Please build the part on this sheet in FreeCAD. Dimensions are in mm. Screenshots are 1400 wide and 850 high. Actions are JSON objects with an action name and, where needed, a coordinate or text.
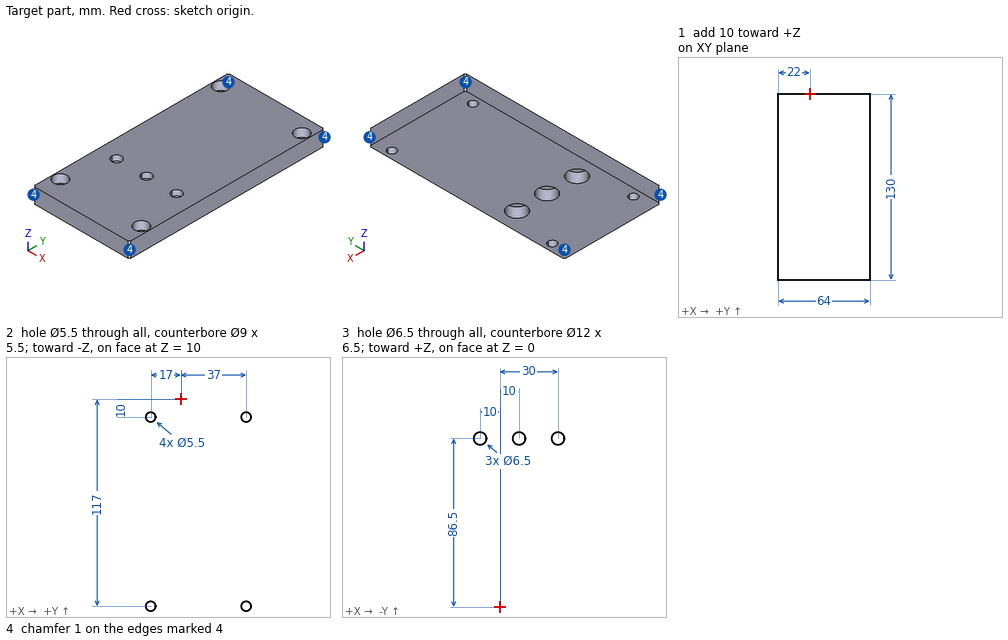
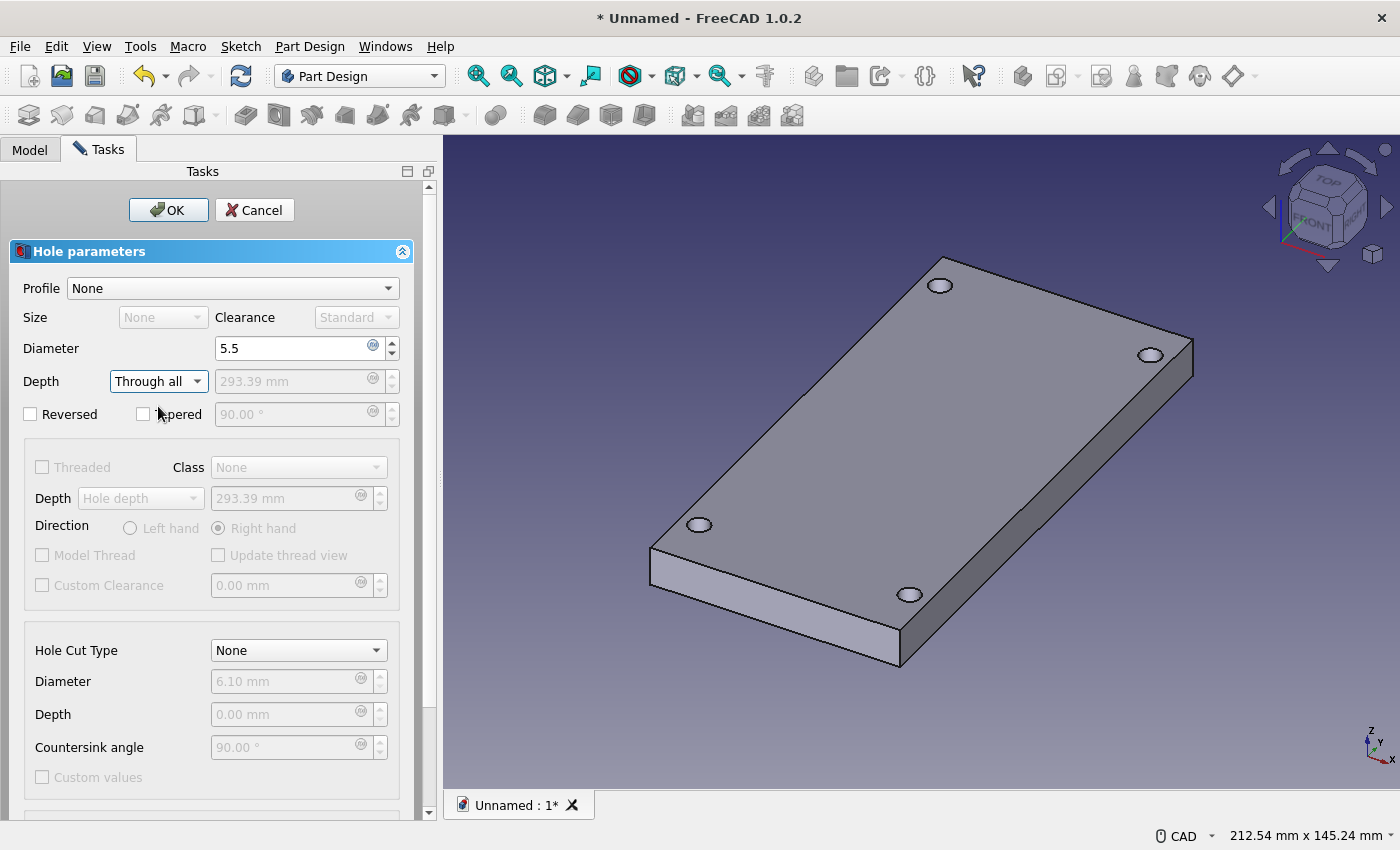
{"action": "left_click", "coordinate": [300, 650]}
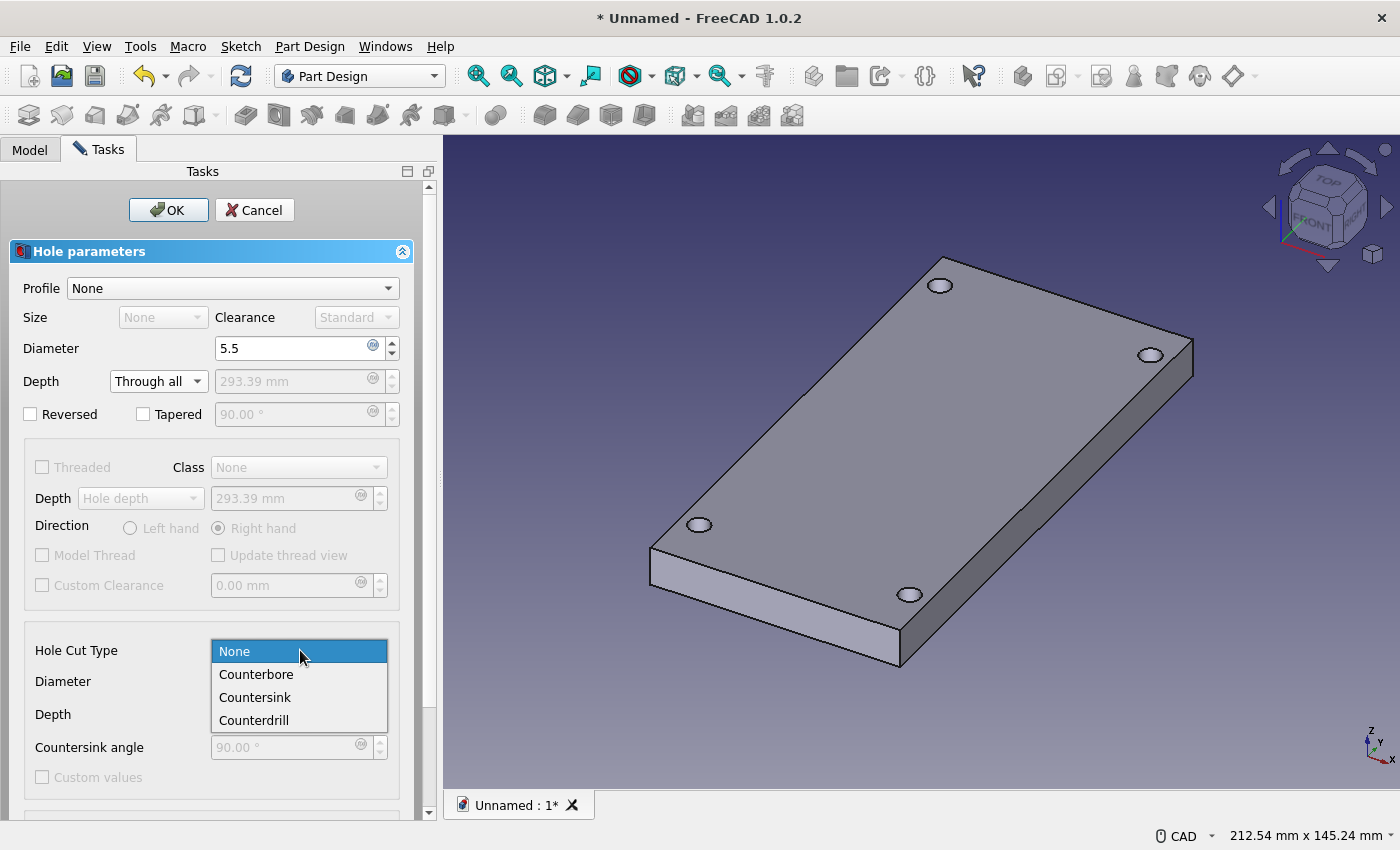
{"action": "left_click", "coordinate": [298, 674]}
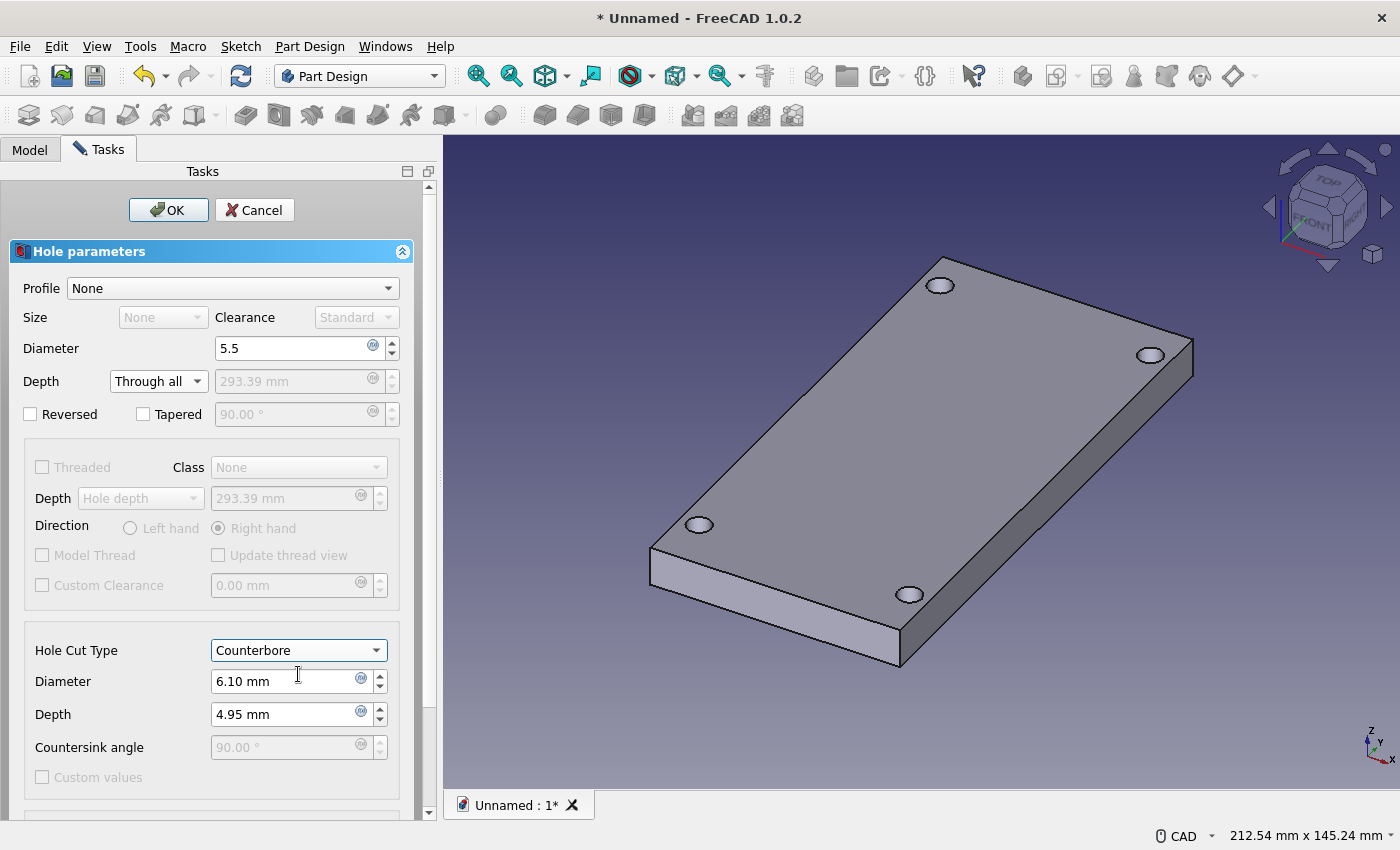
{"action": "triple_click", "coordinate": [292, 682]}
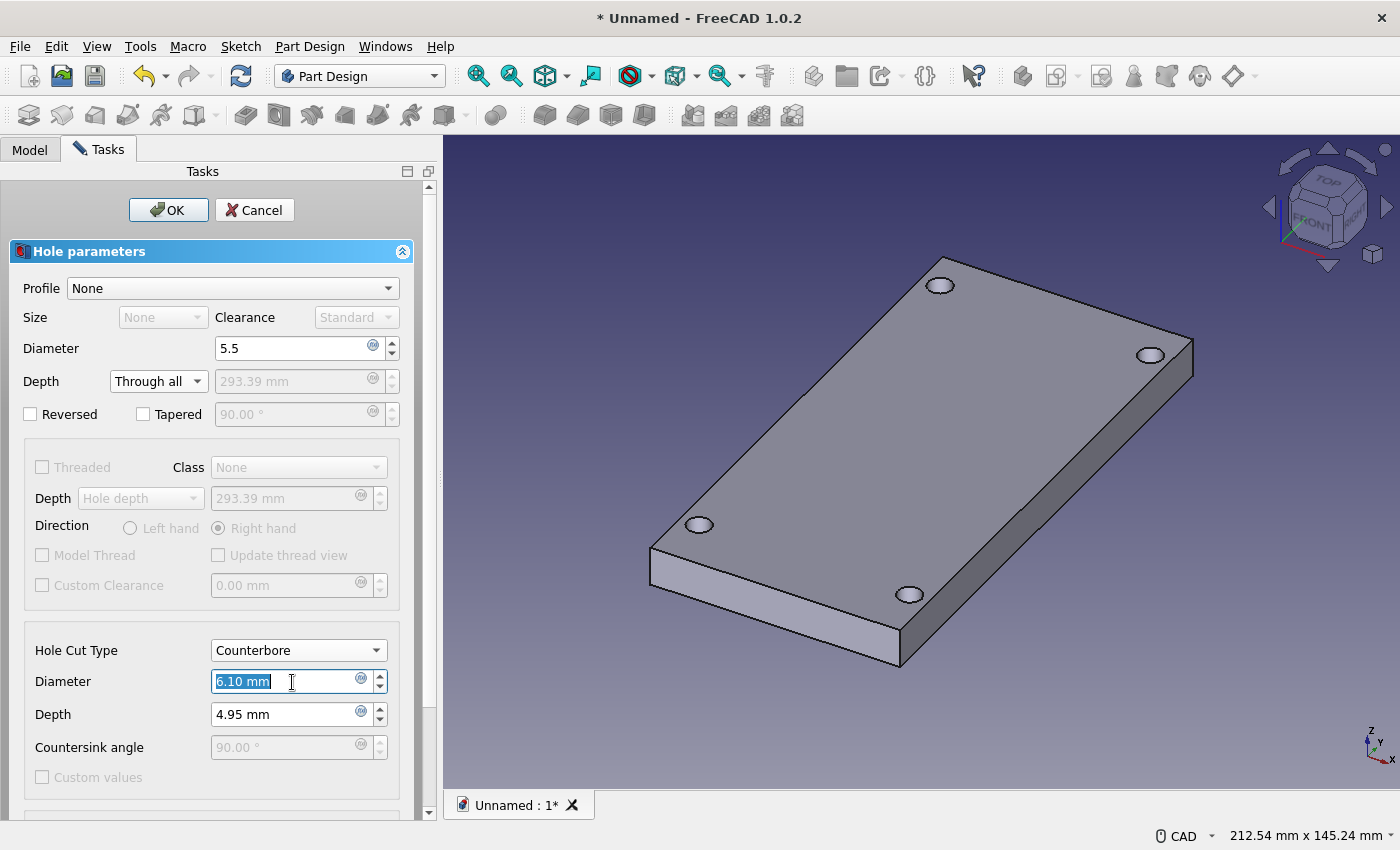
{"action": "type", "text": "9"}
{"action": "key", "text": "Tab"}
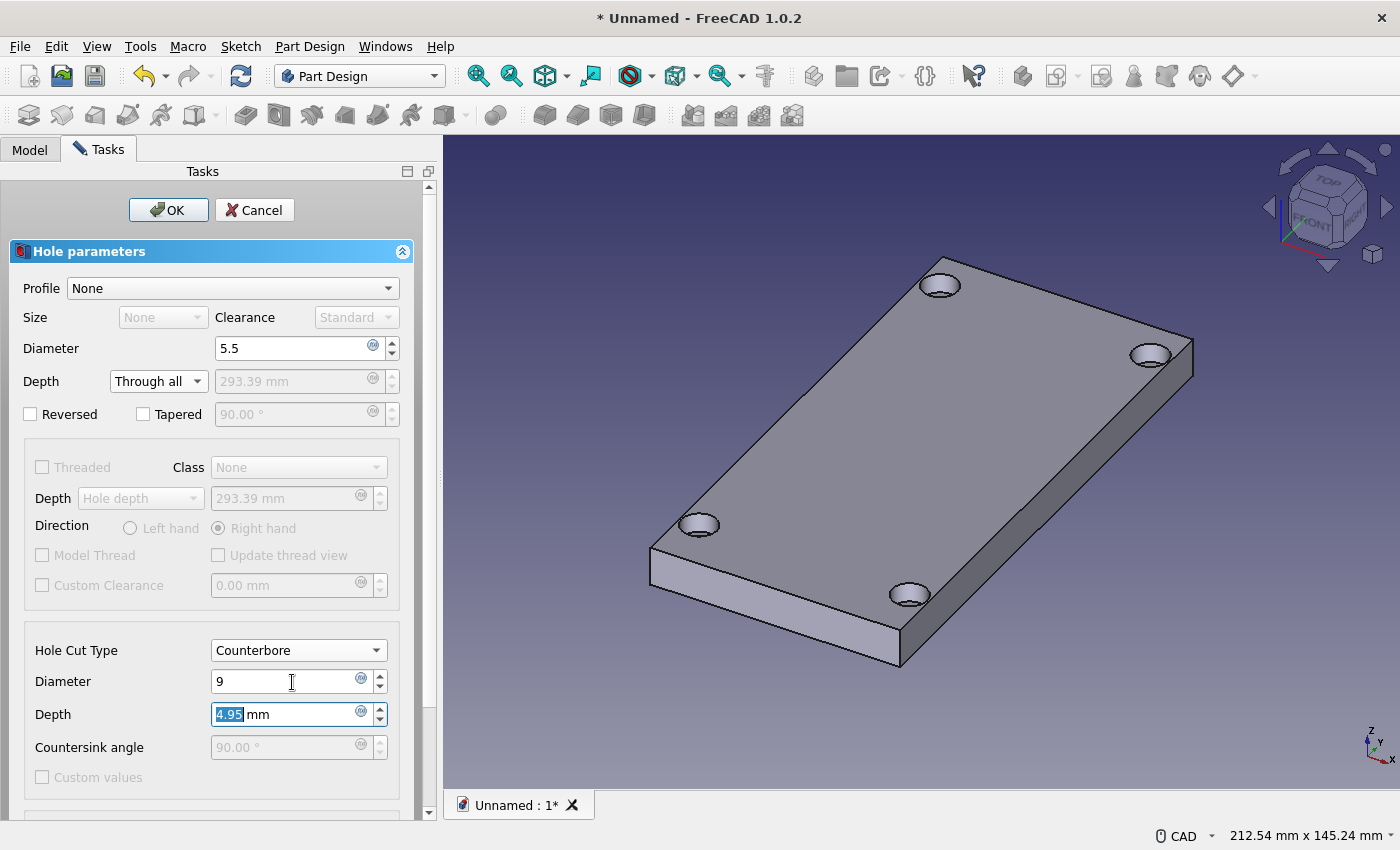
{"action": "type", "text": "5.5"}
{"action": "key", "text": "Tab"}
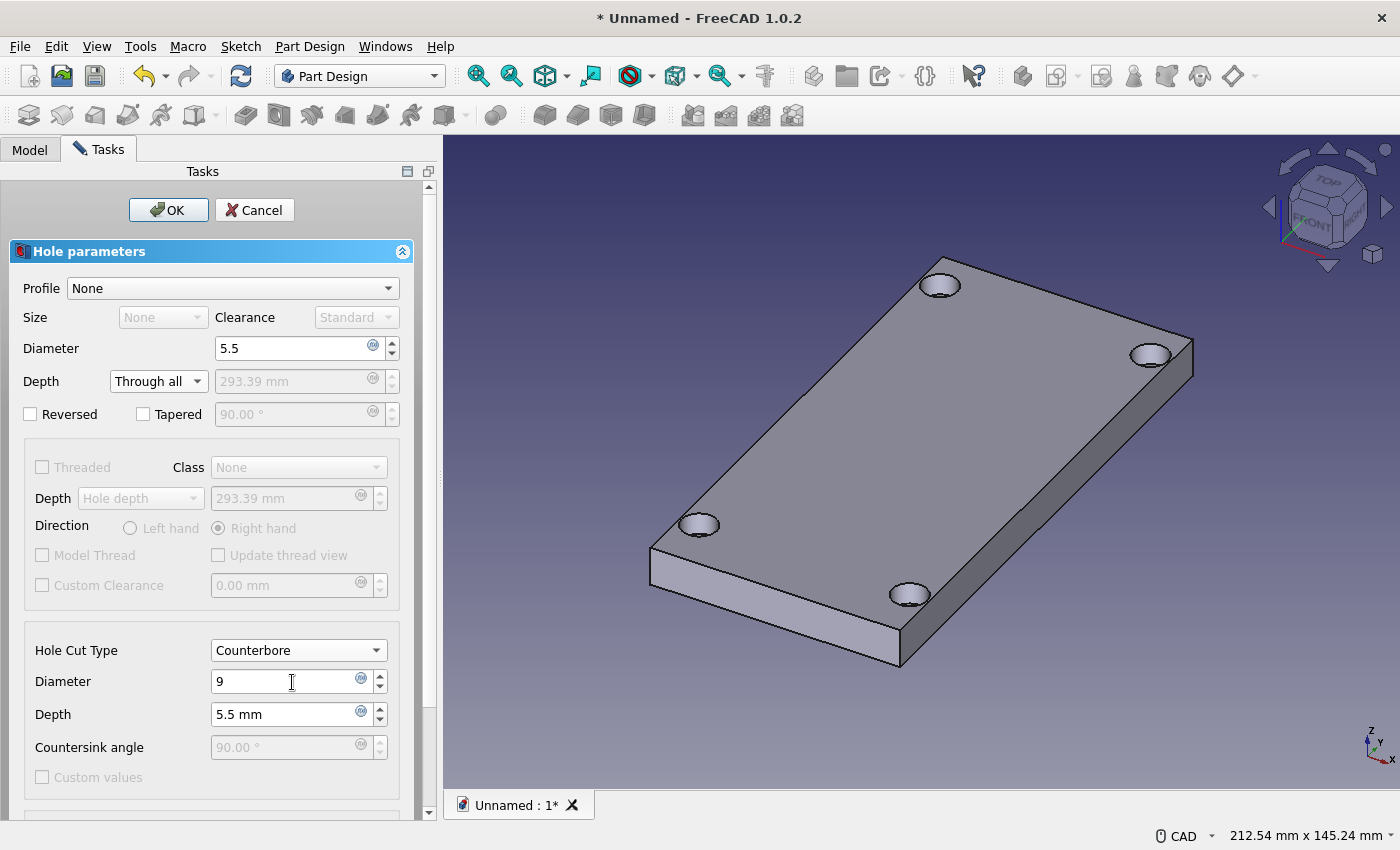
{"action": "left_click", "coordinate": [169, 210]}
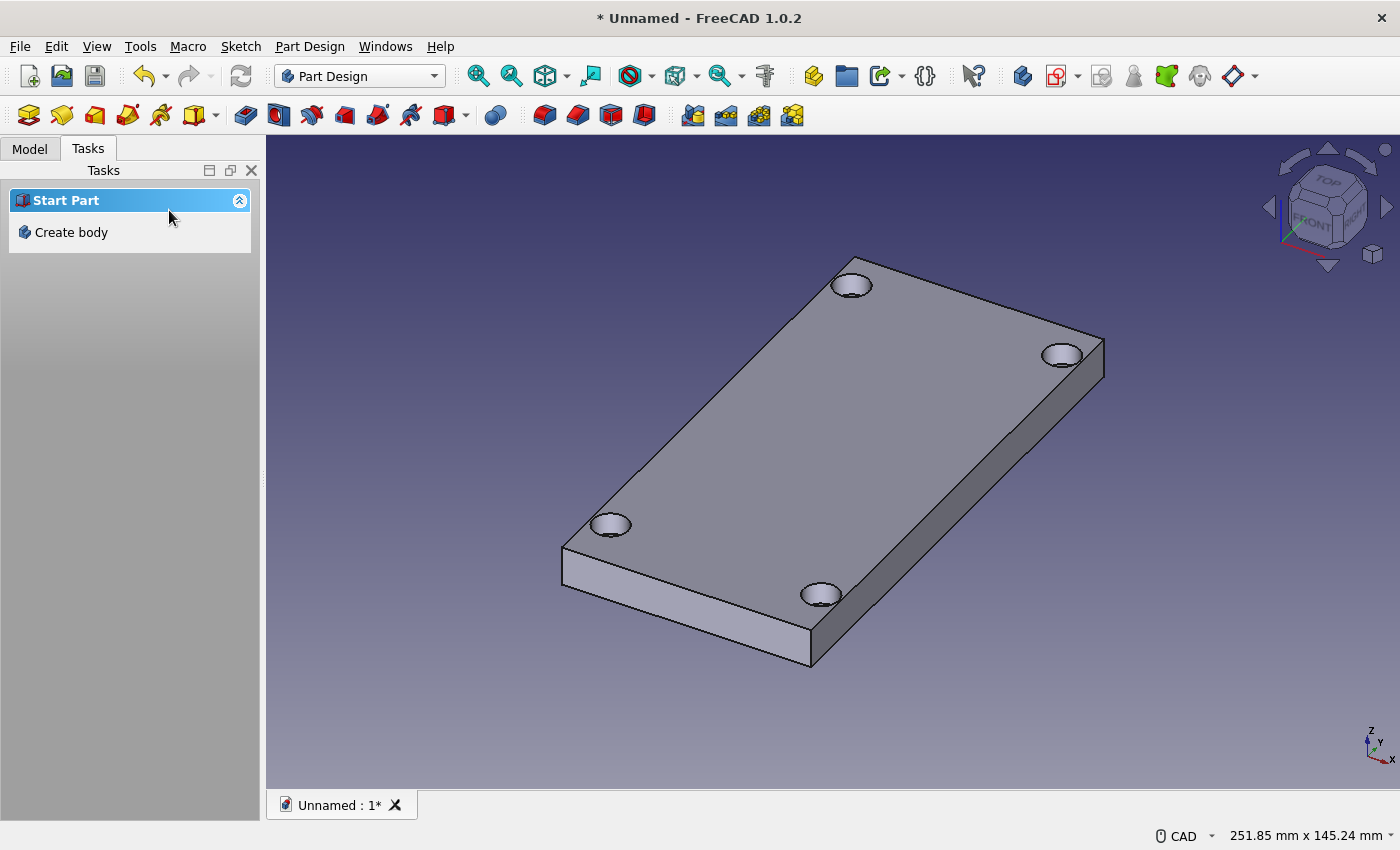
{"action": "key", "text": "5"}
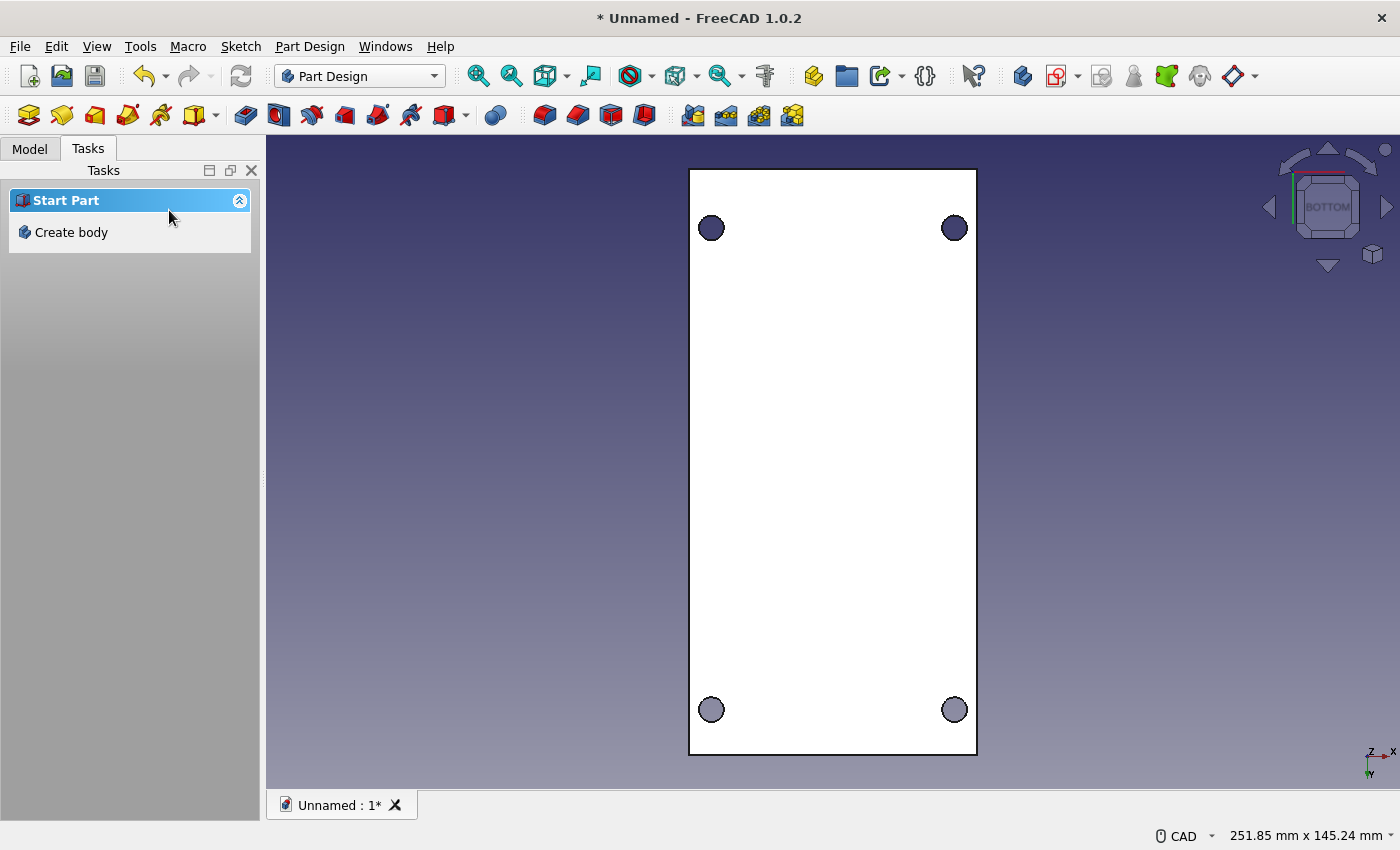
{"action": "left_click", "coordinate": [833, 545]}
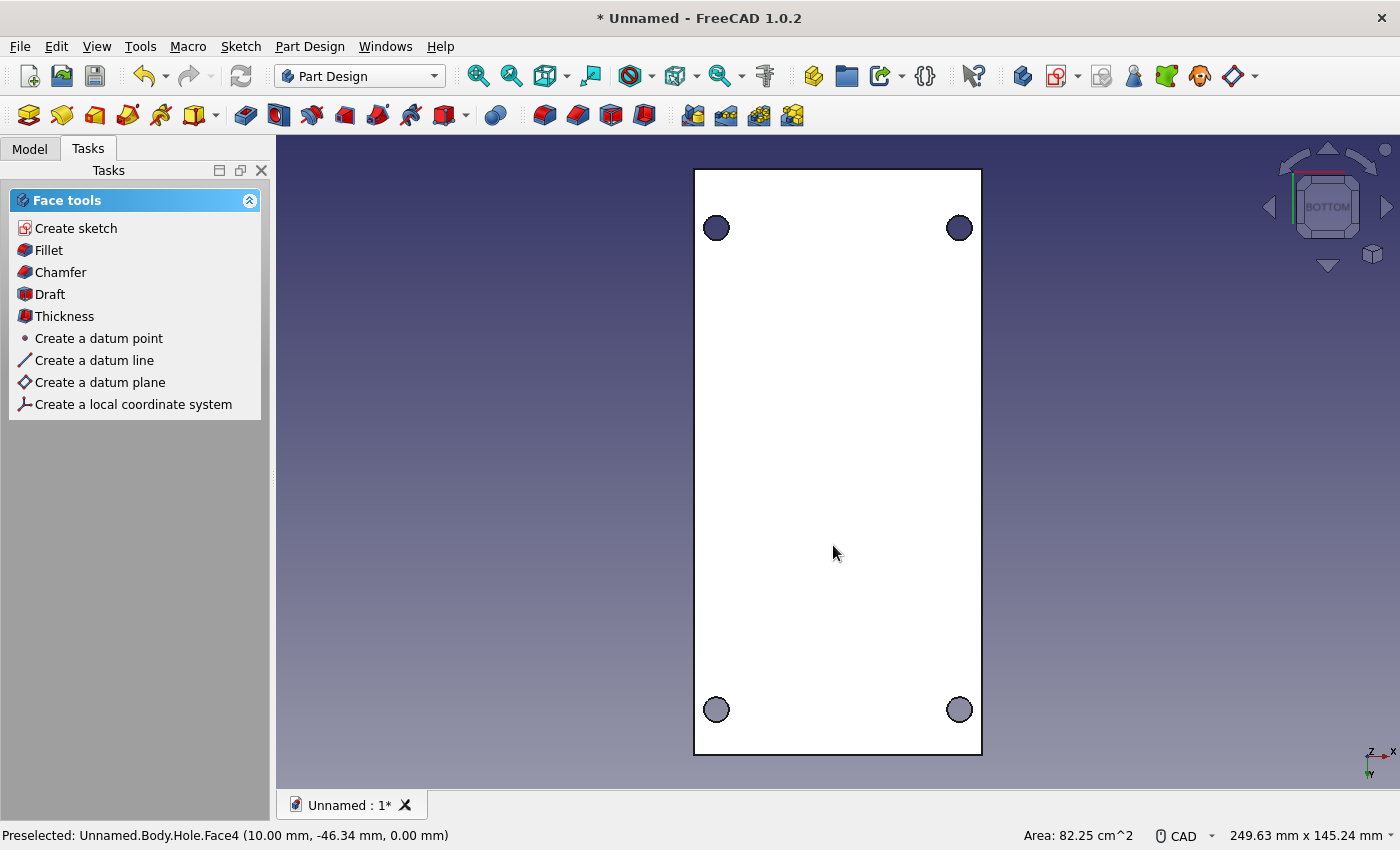
{"action": "left_click", "coordinate": [1056, 76]}